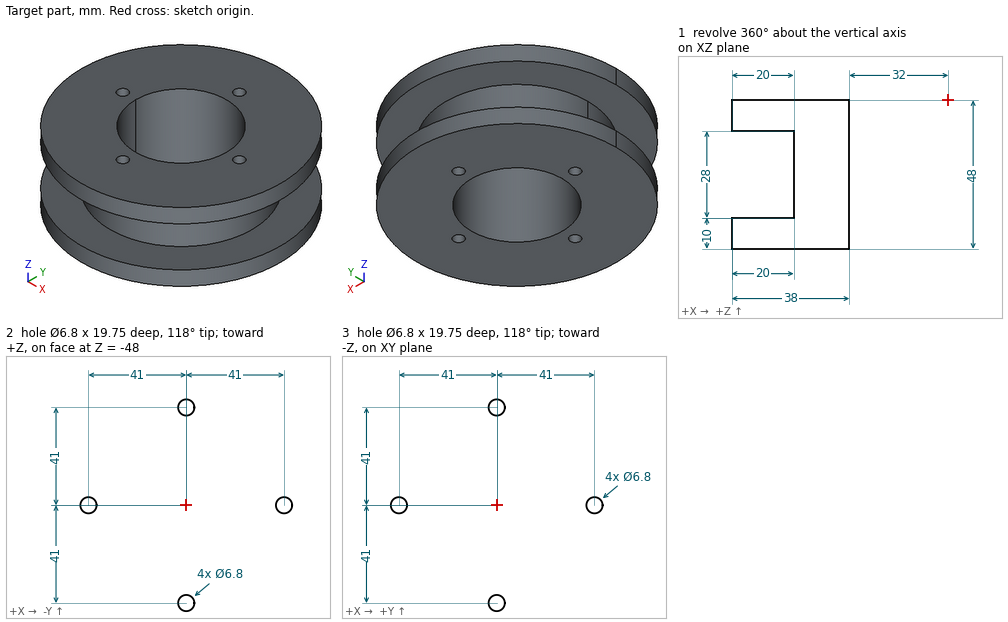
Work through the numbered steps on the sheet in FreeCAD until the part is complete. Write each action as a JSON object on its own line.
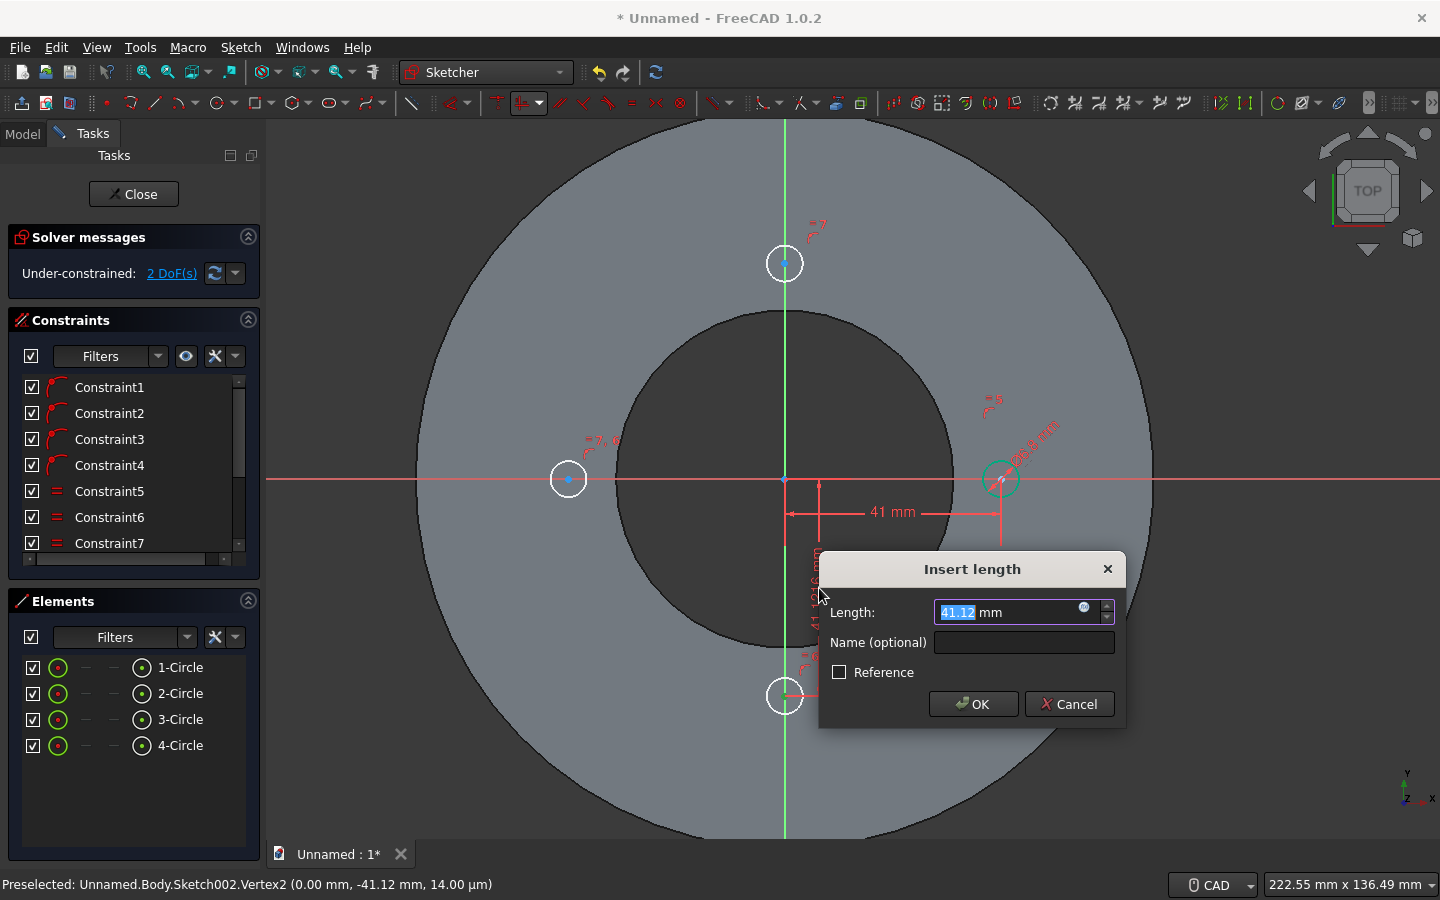
{"action": "type", "text": "41"}
{"action": "key", "text": "Return"}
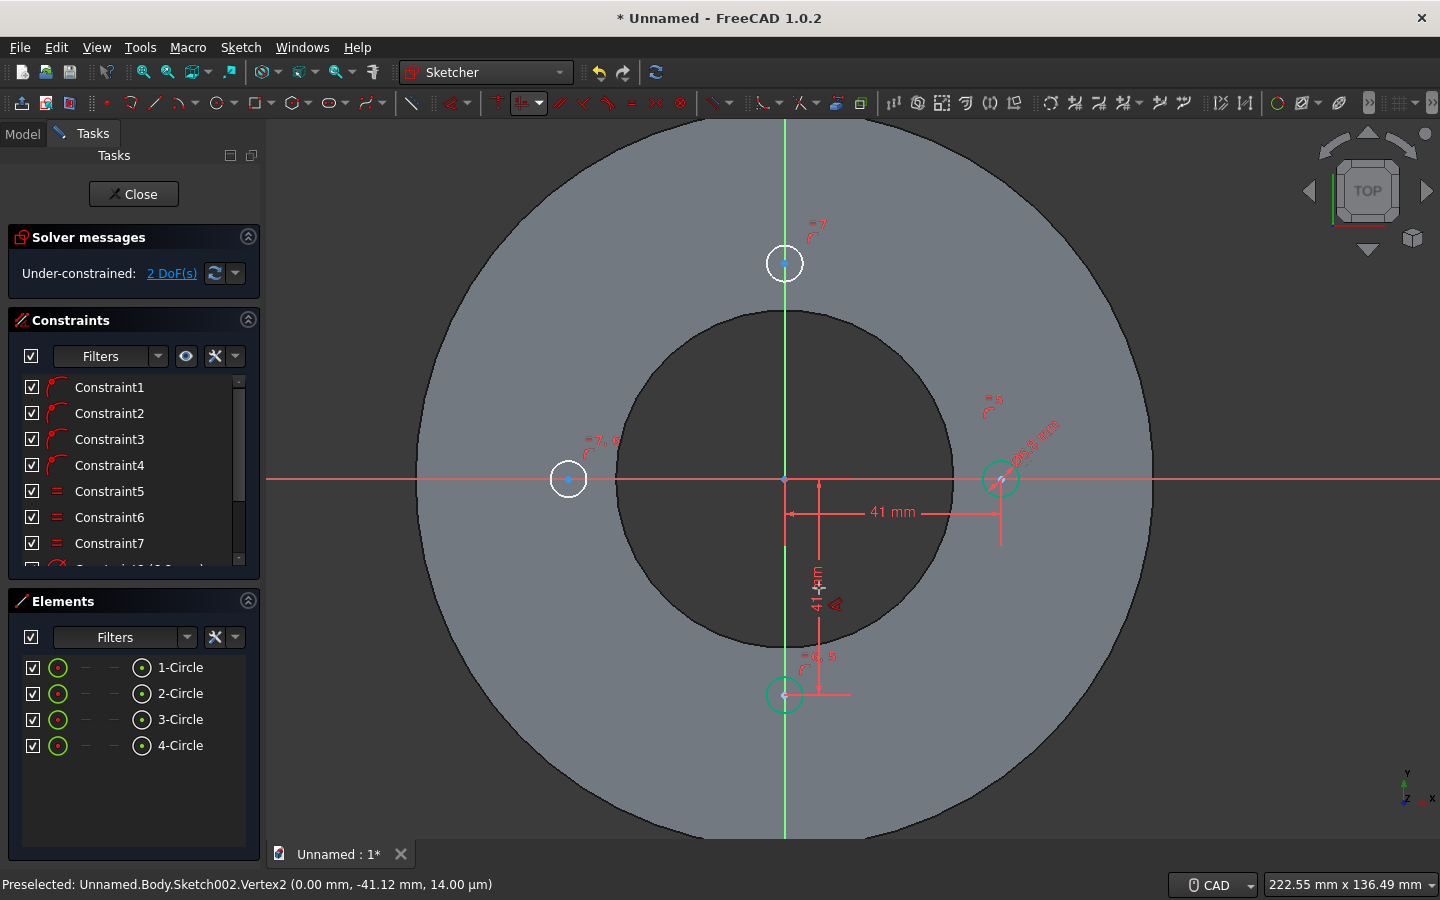
{"action": "left_click", "coordinate": [569, 479]}
{"action": "left_click", "coordinate": [677, 513]}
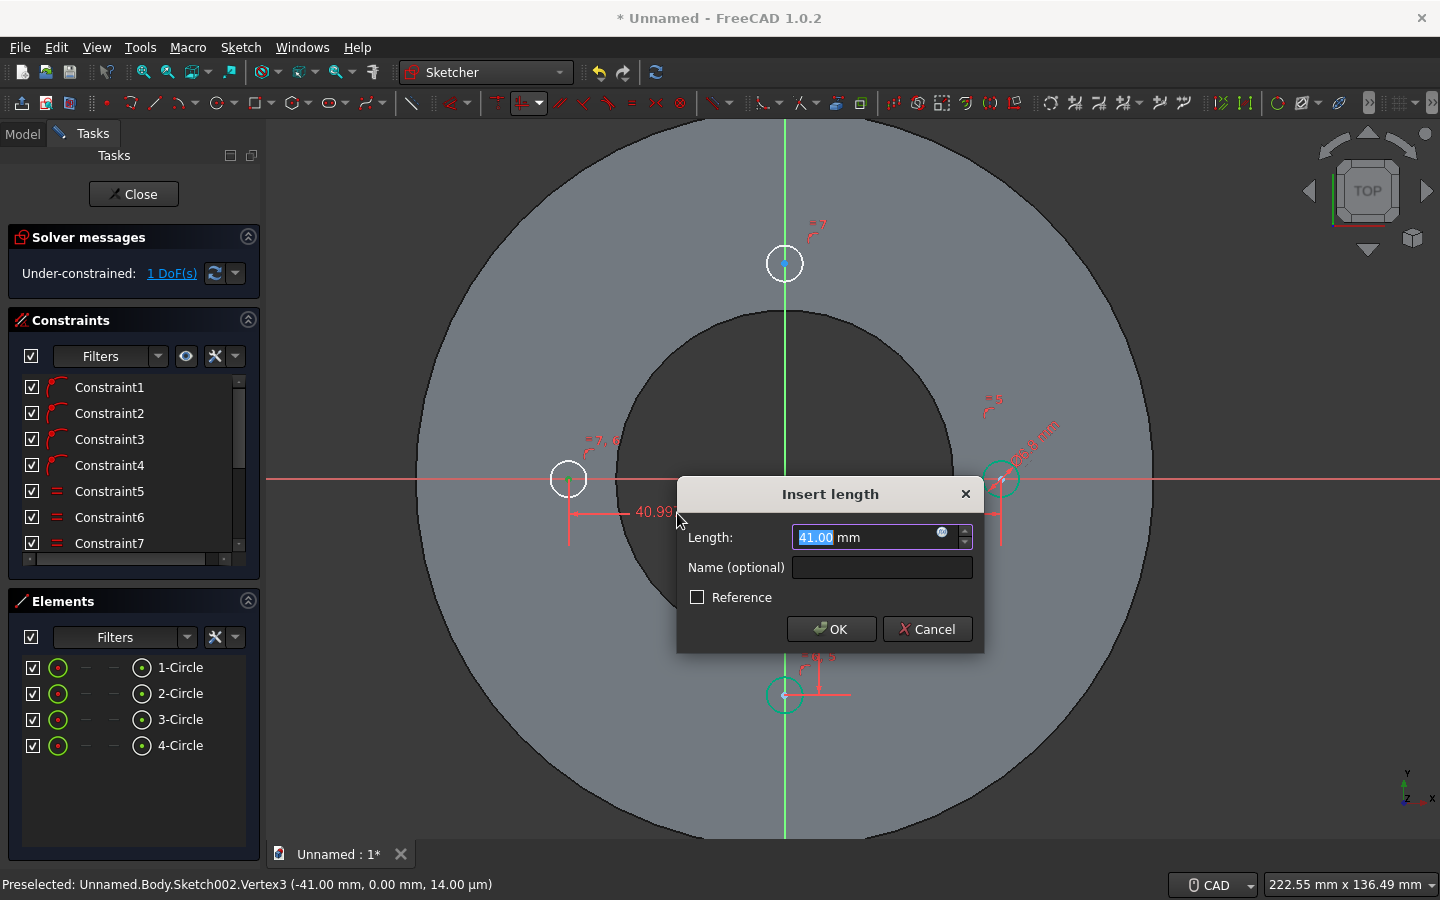
{"action": "type", "text": "41"}
{"action": "key", "text": "Return"}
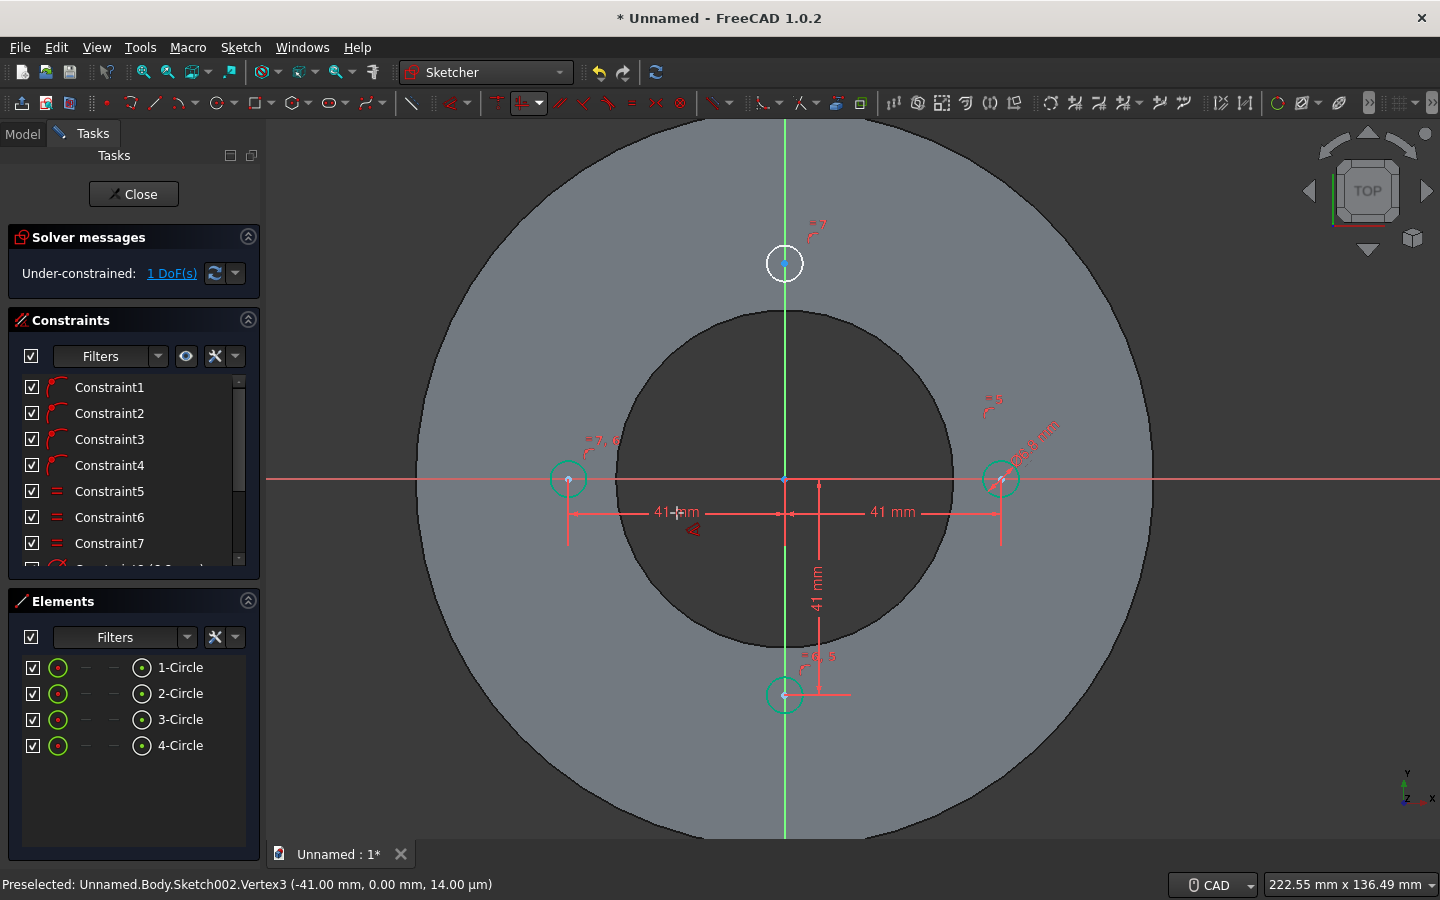
{"action": "left_click", "coordinate": [785, 264]}
{"action": "left_click", "coordinate": [819, 371]}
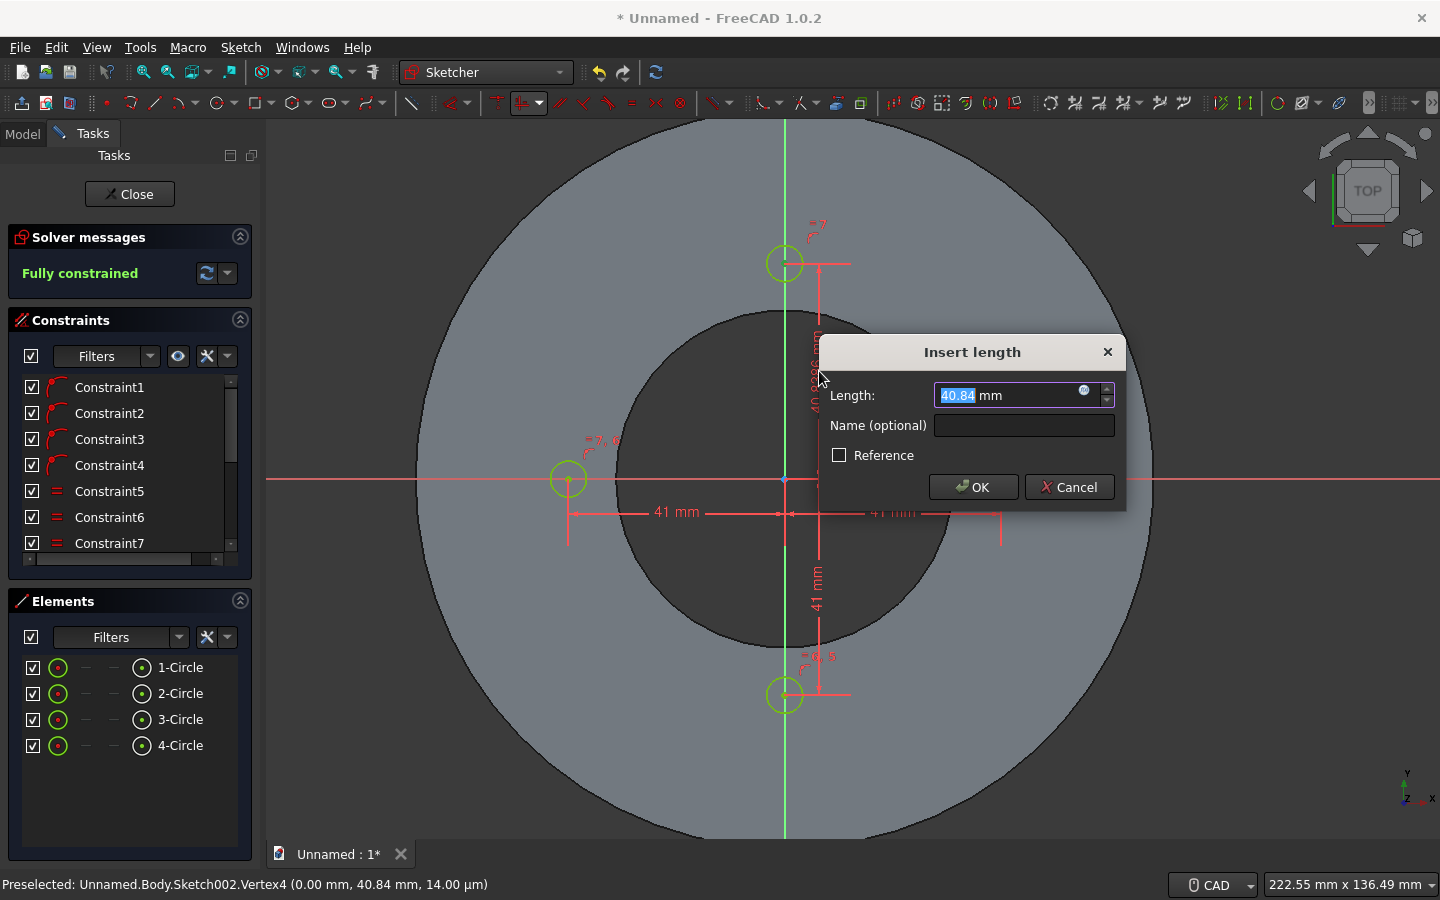
{"action": "type", "text": "41"}
{"action": "key", "text": "Return"}
{"action": "key", "text": "Escape"}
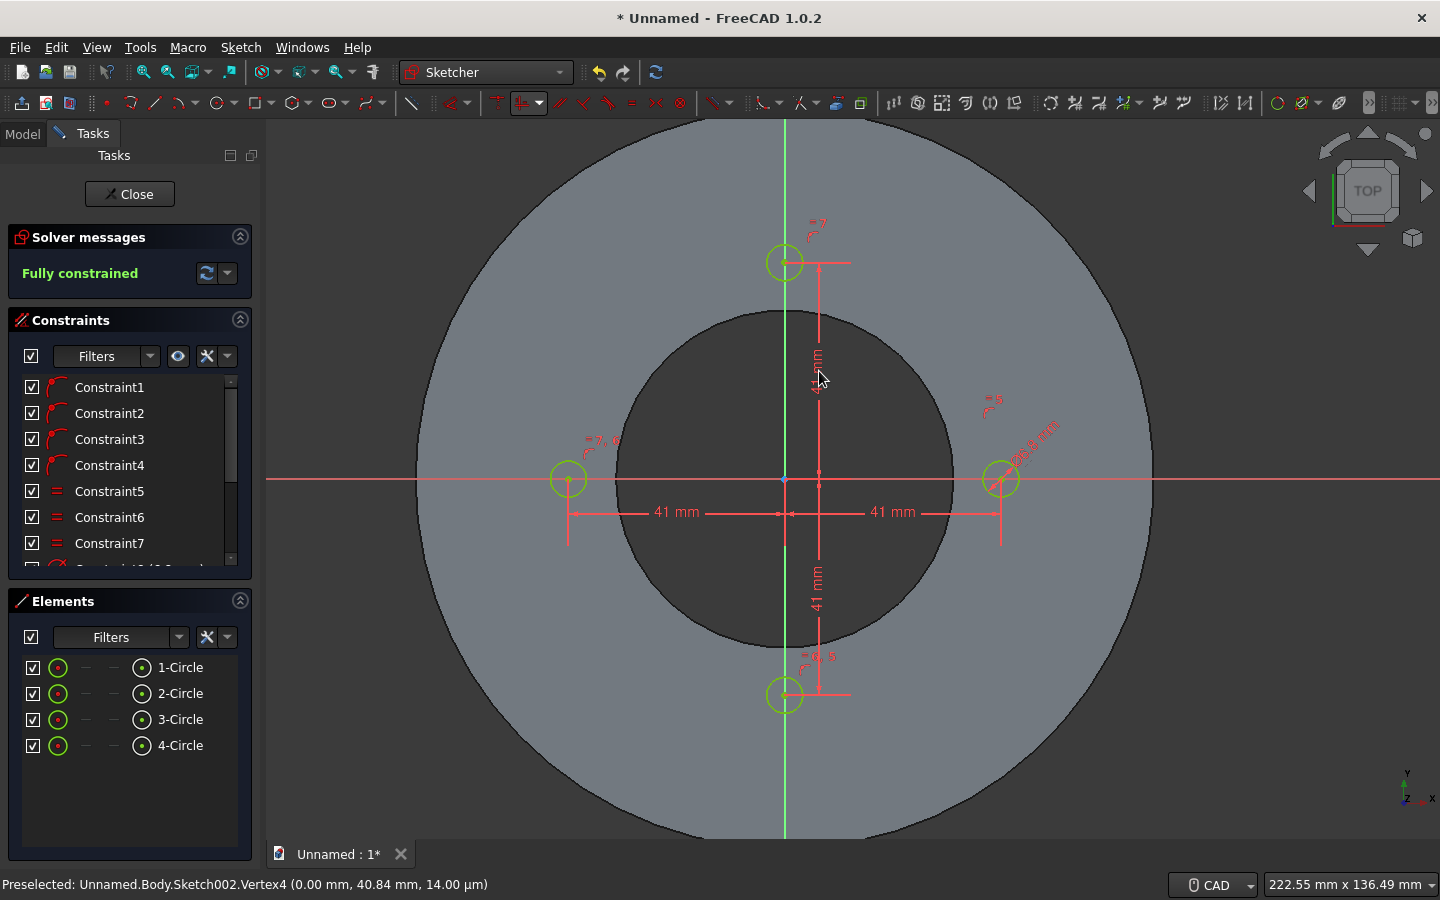
{"action": "left_click", "coordinate": [130, 194]}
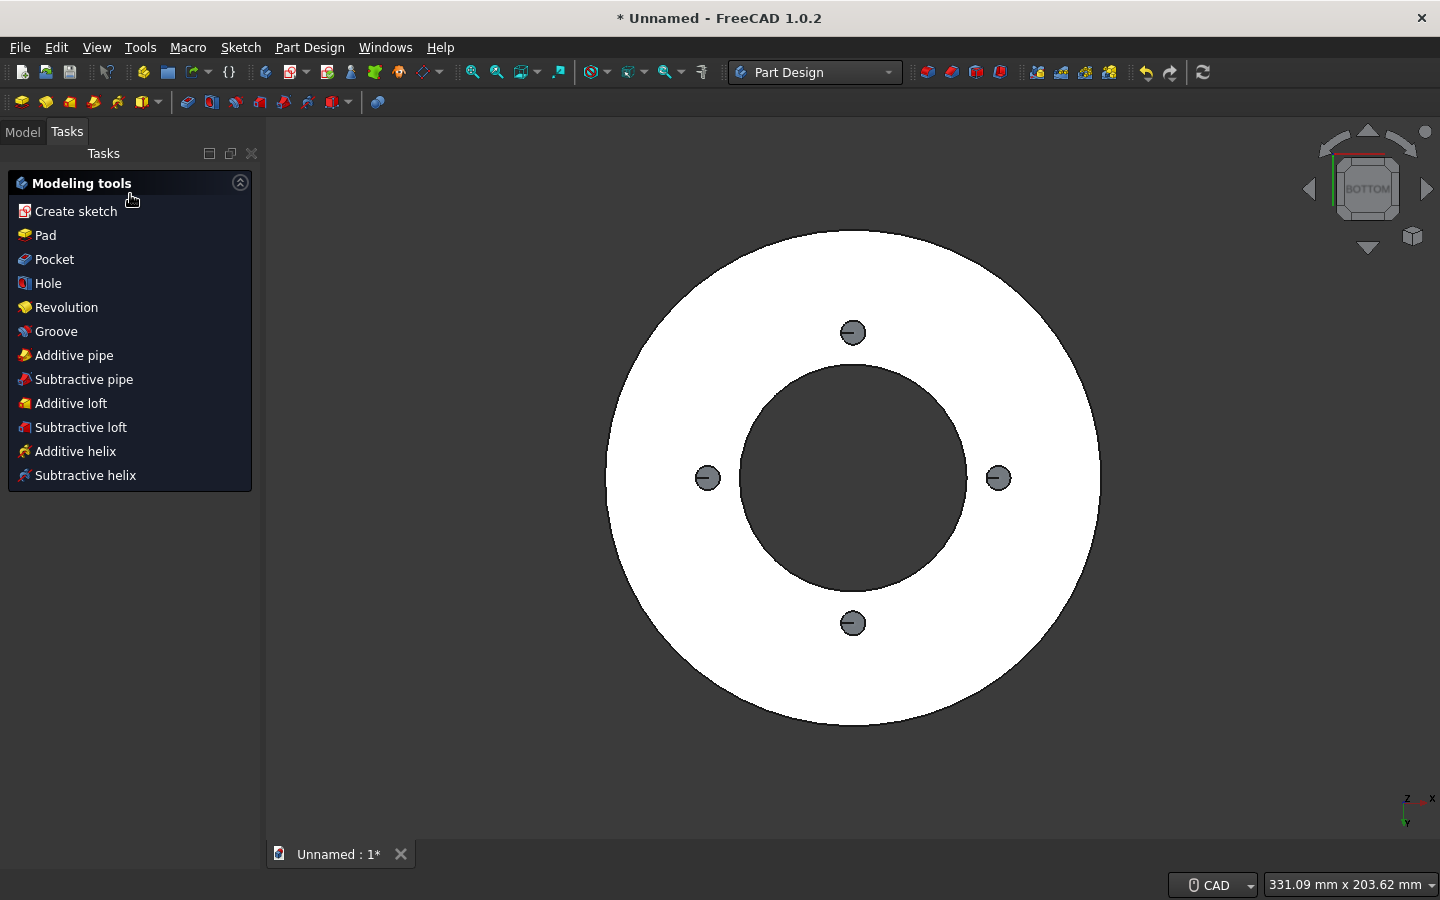
{"action": "left_click", "coordinate": [212, 102]}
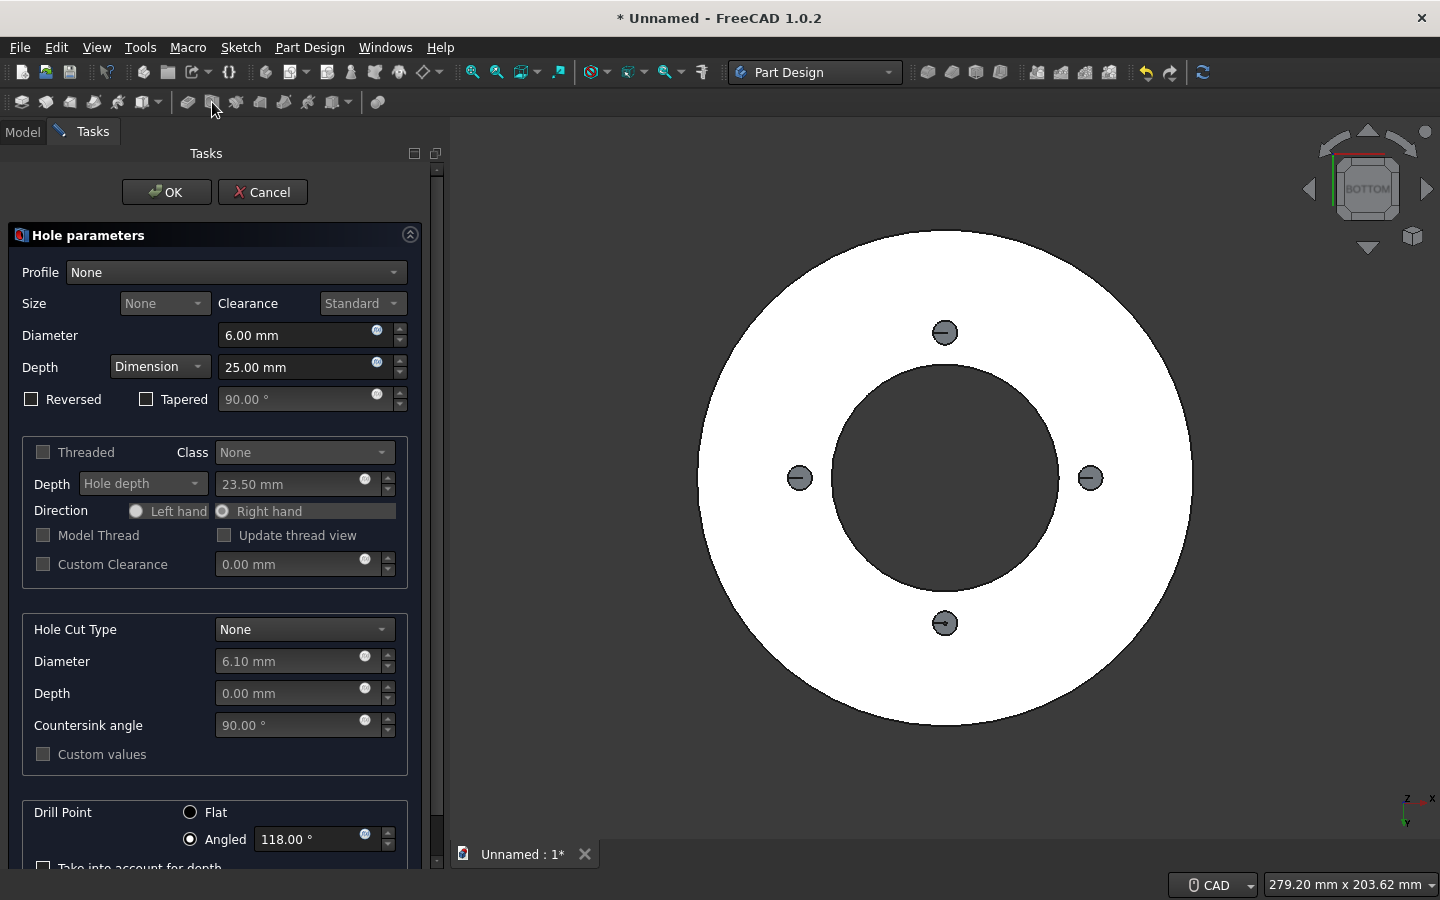
{"action": "triple_click", "coordinate": [305, 335]}